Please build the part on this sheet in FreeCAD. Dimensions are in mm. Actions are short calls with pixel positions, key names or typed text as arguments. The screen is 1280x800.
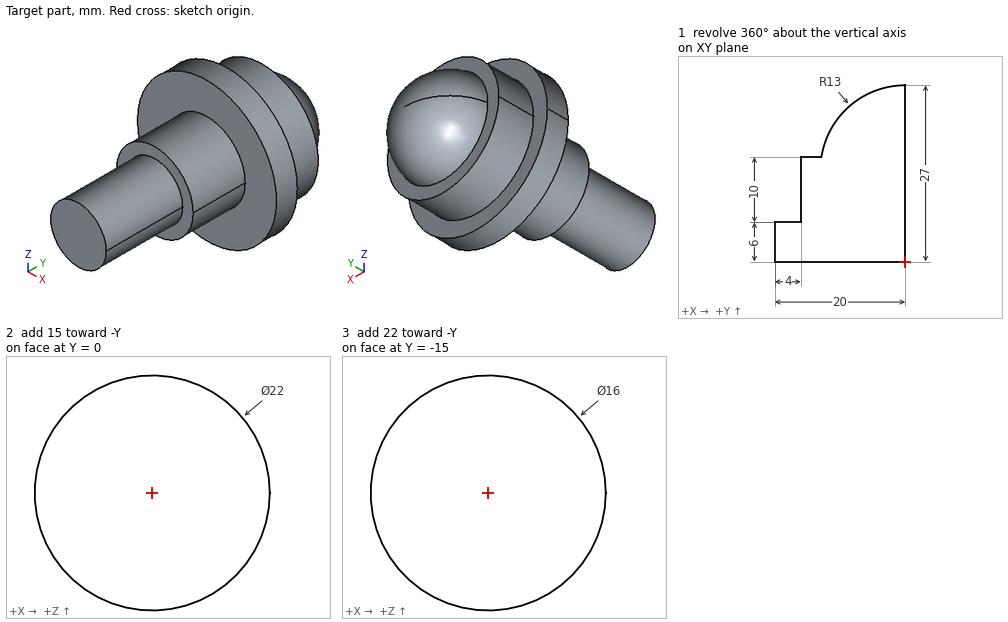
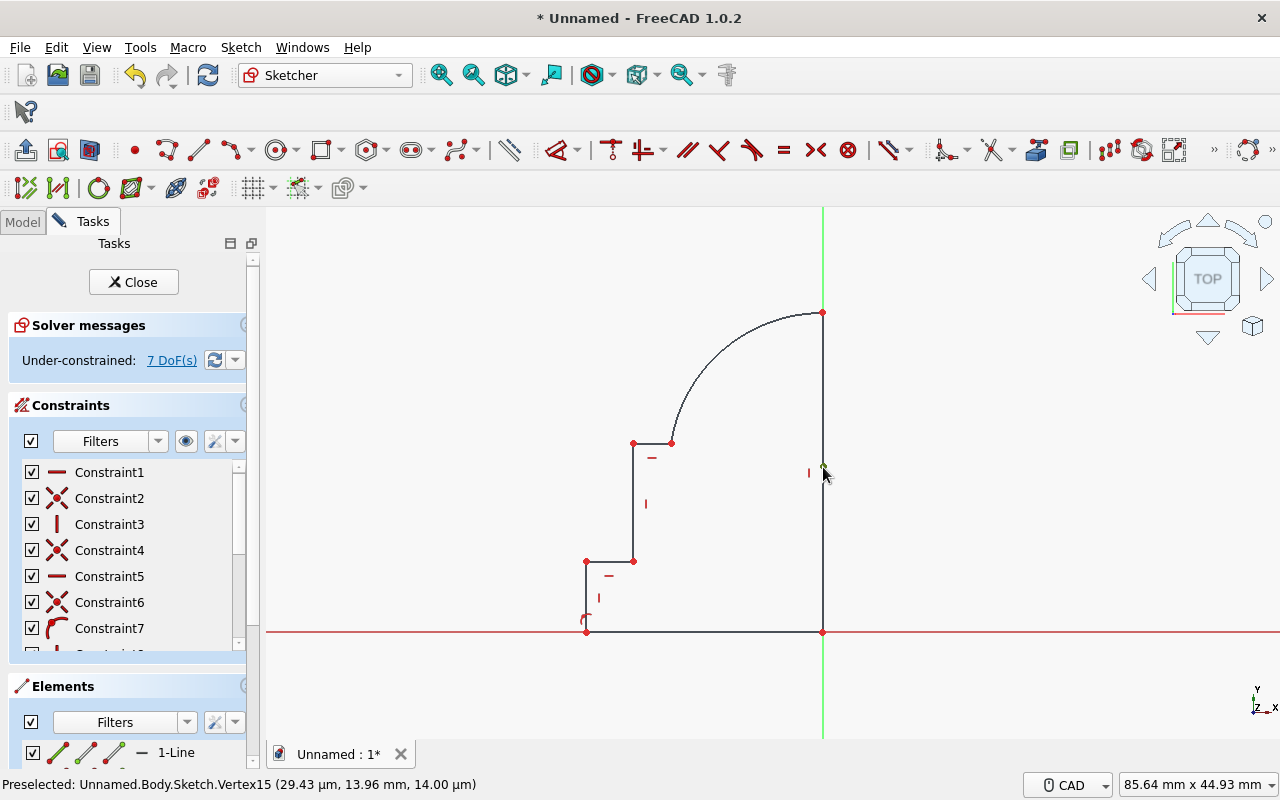
click(823, 677)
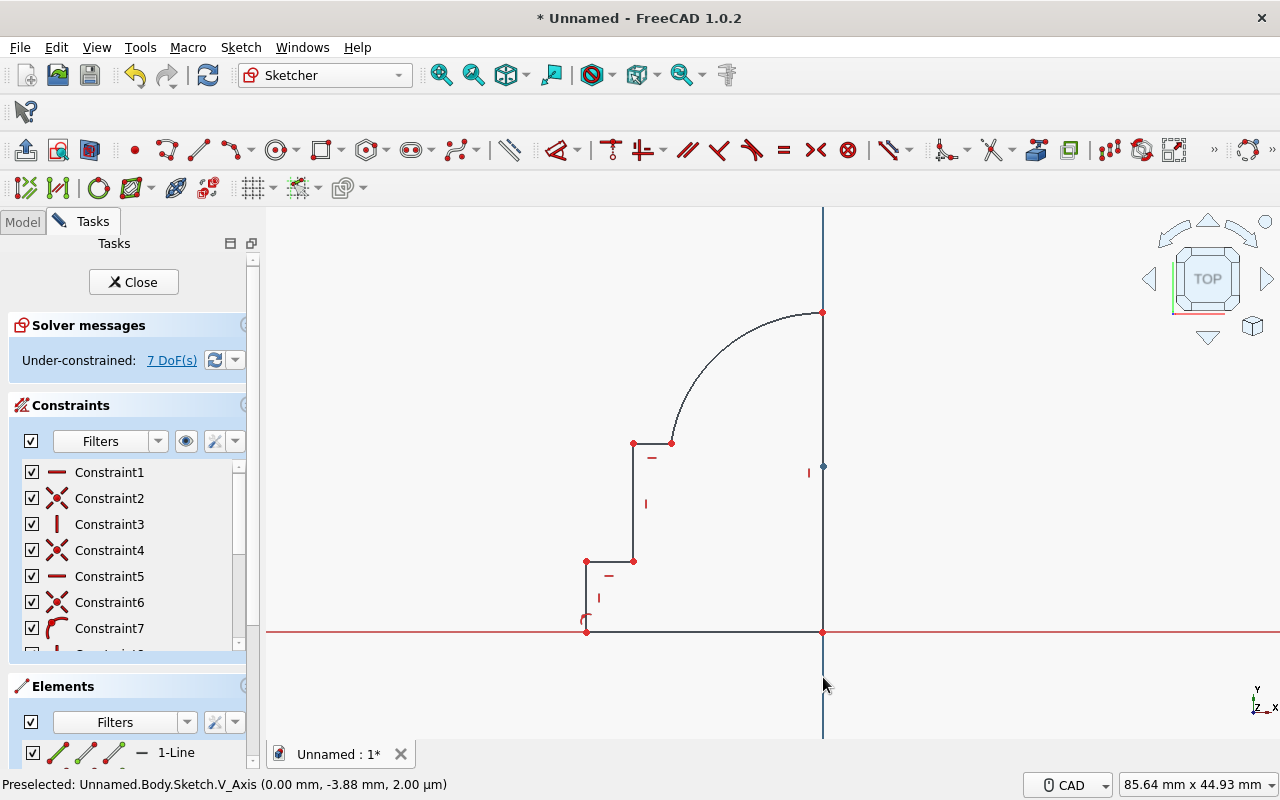
click(612, 150)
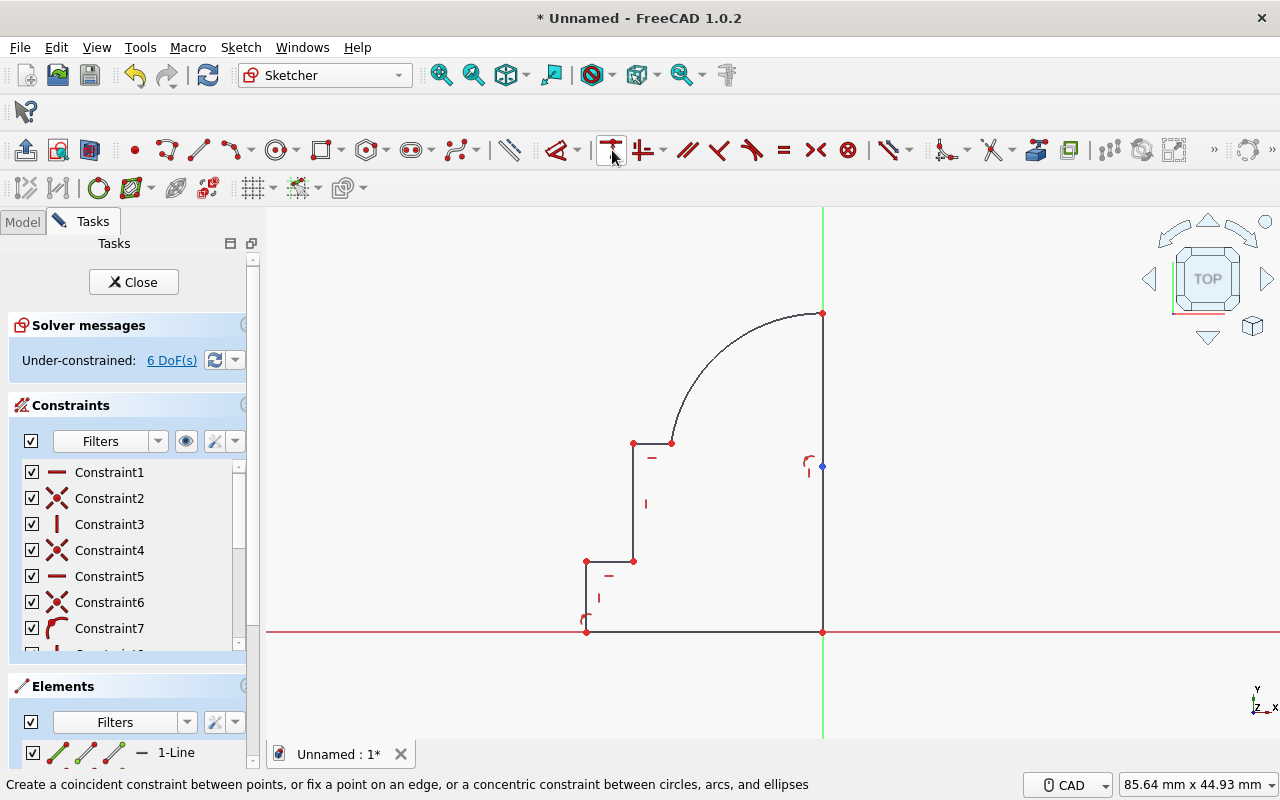
click(556, 150)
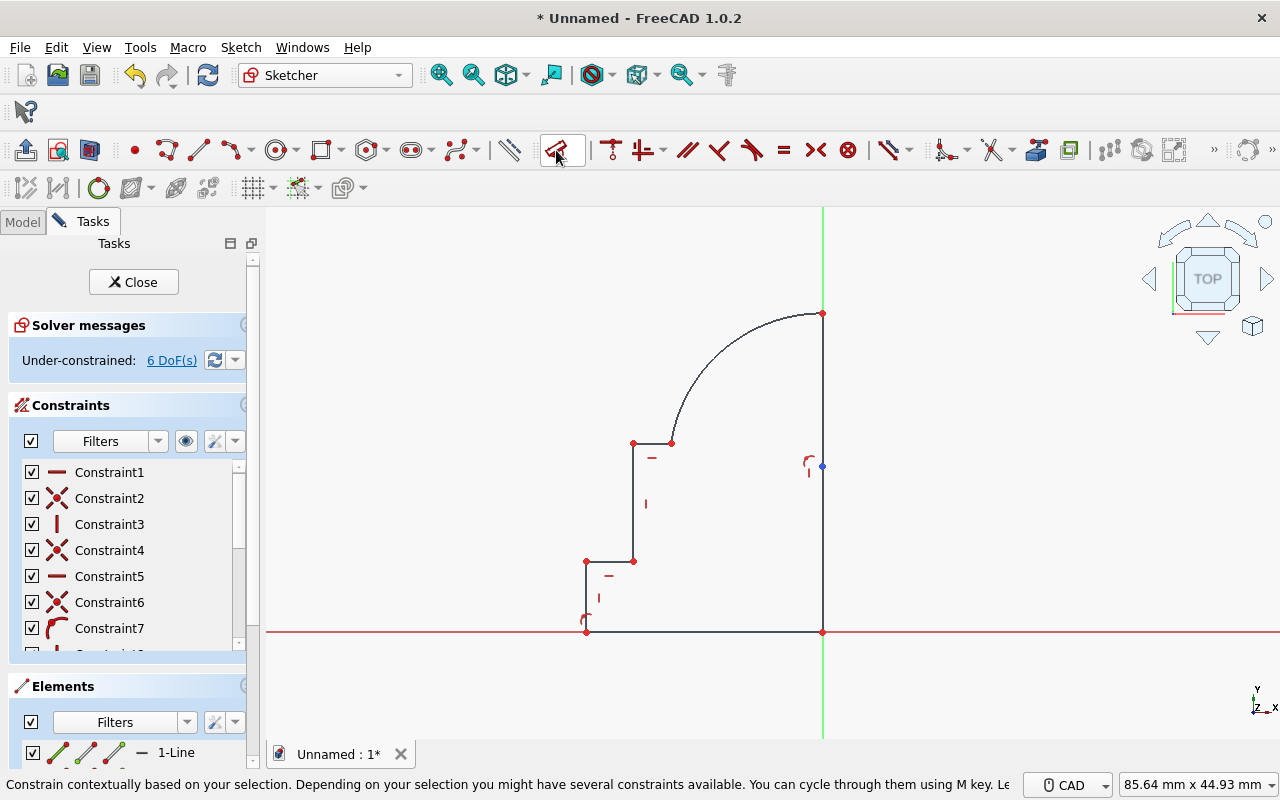
click(759, 327)
click(746, 298)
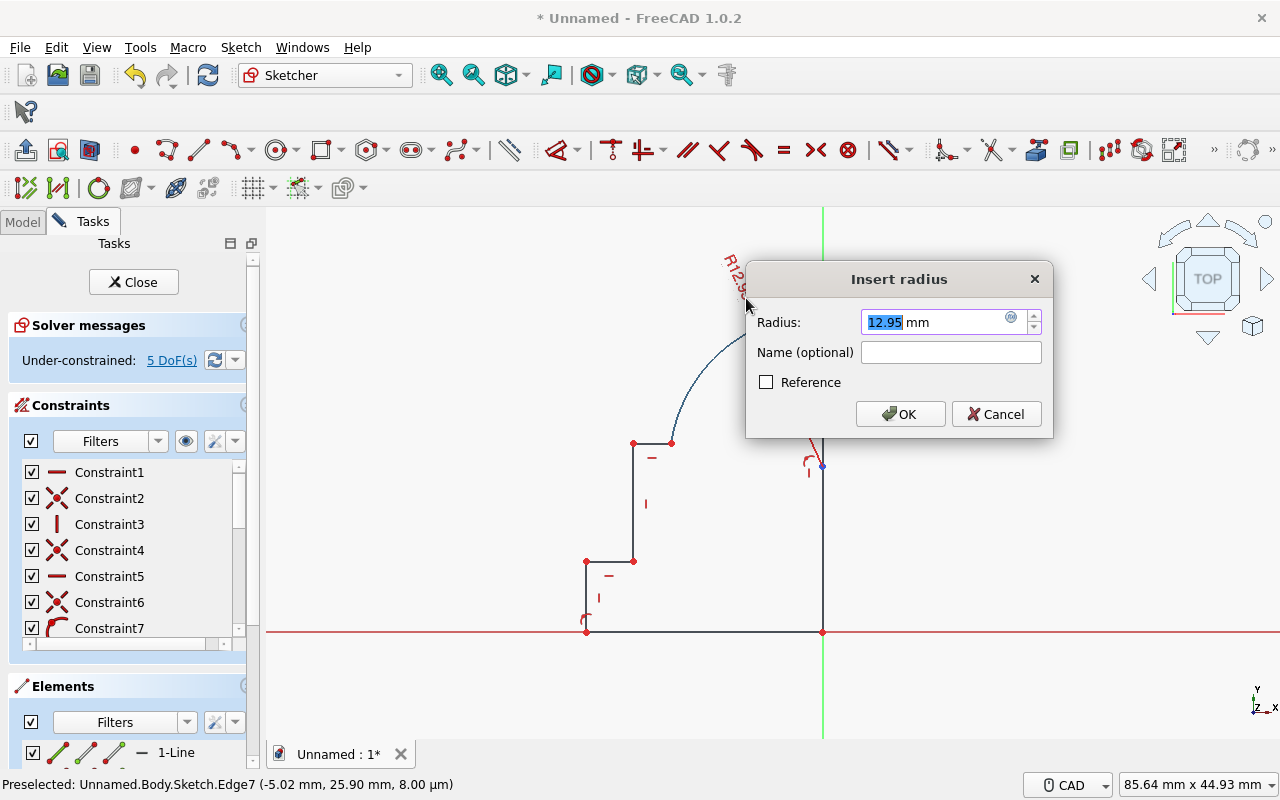
text(13)
key(Return)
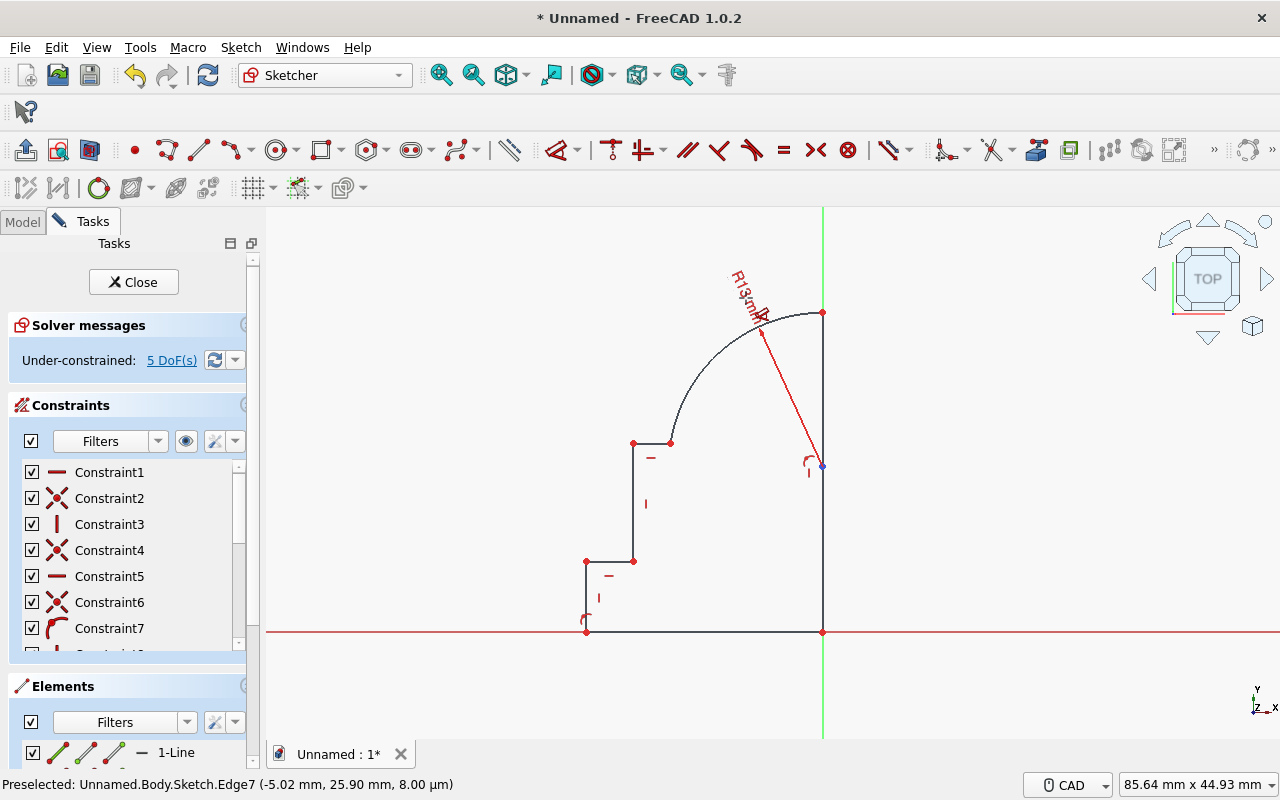
click(619, 562)
click(609, 596)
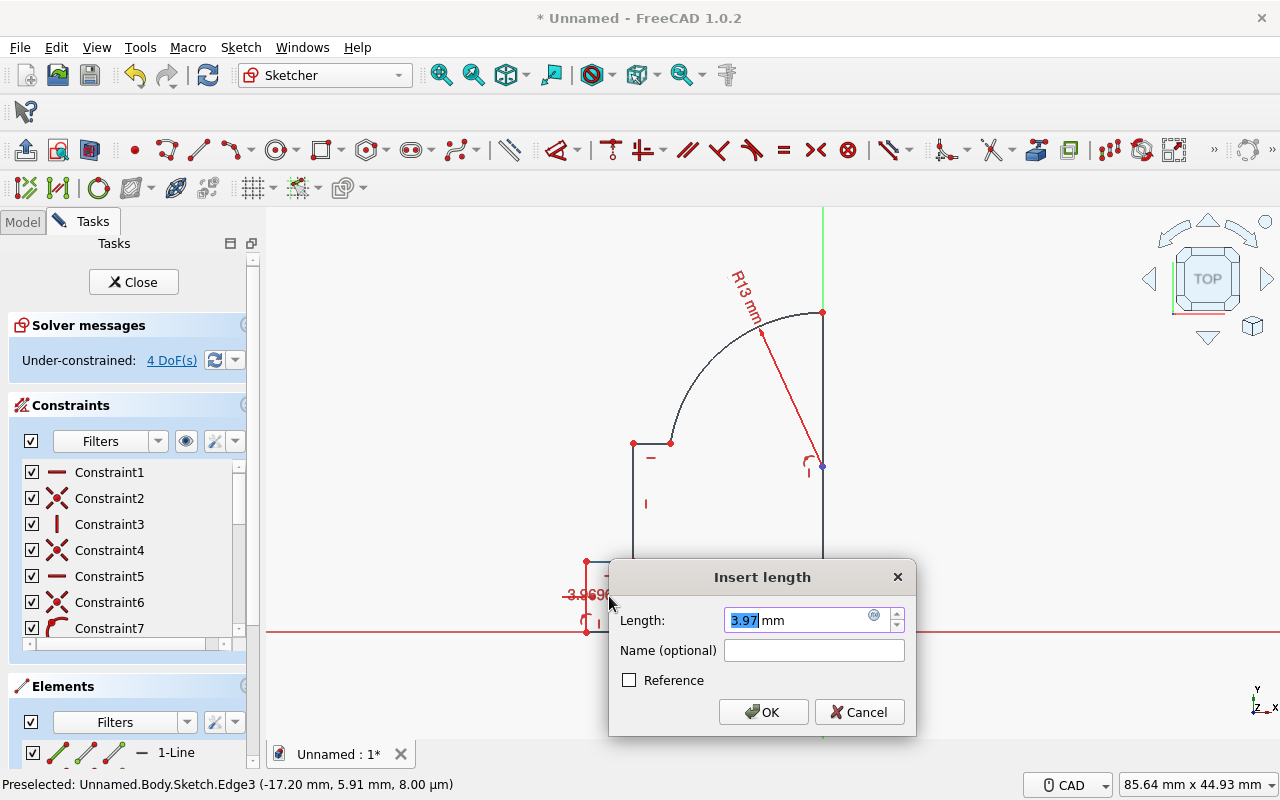
text(4)
key(Return)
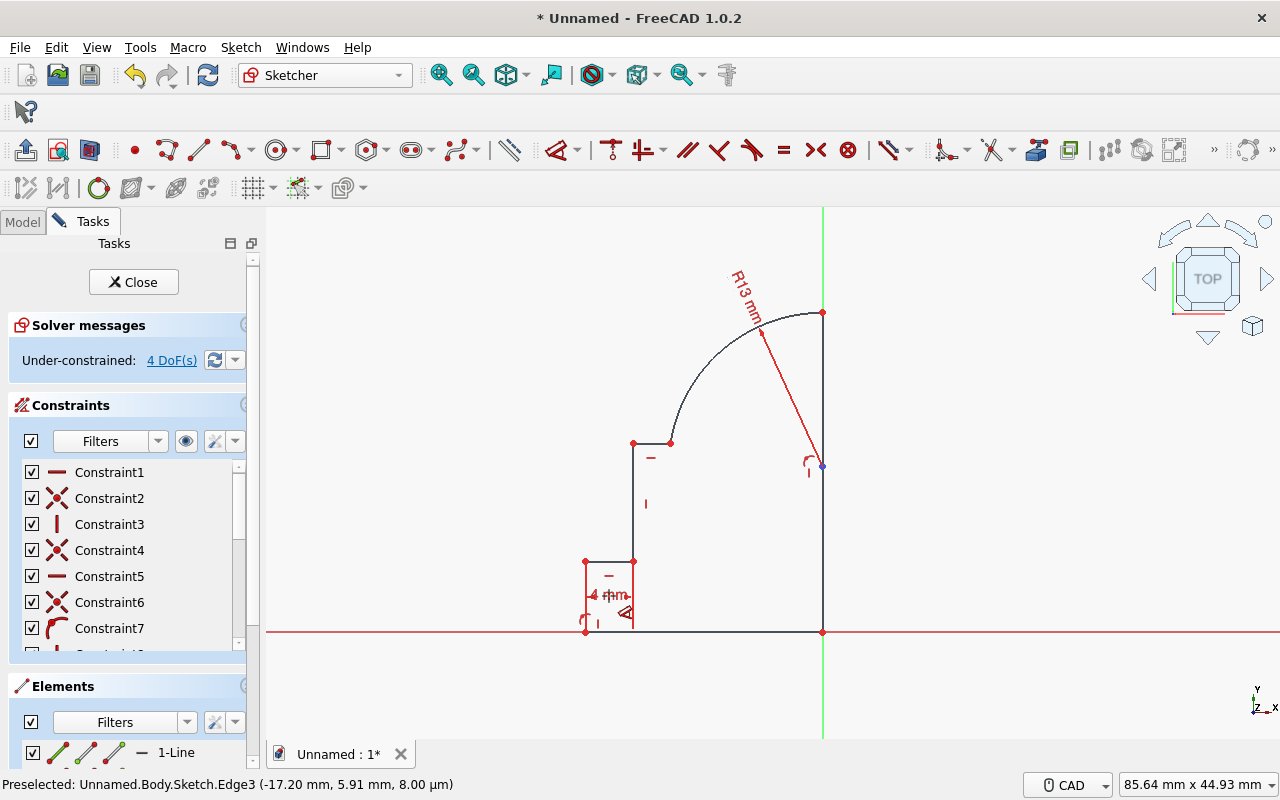
click(586, 583)
click(552, 573)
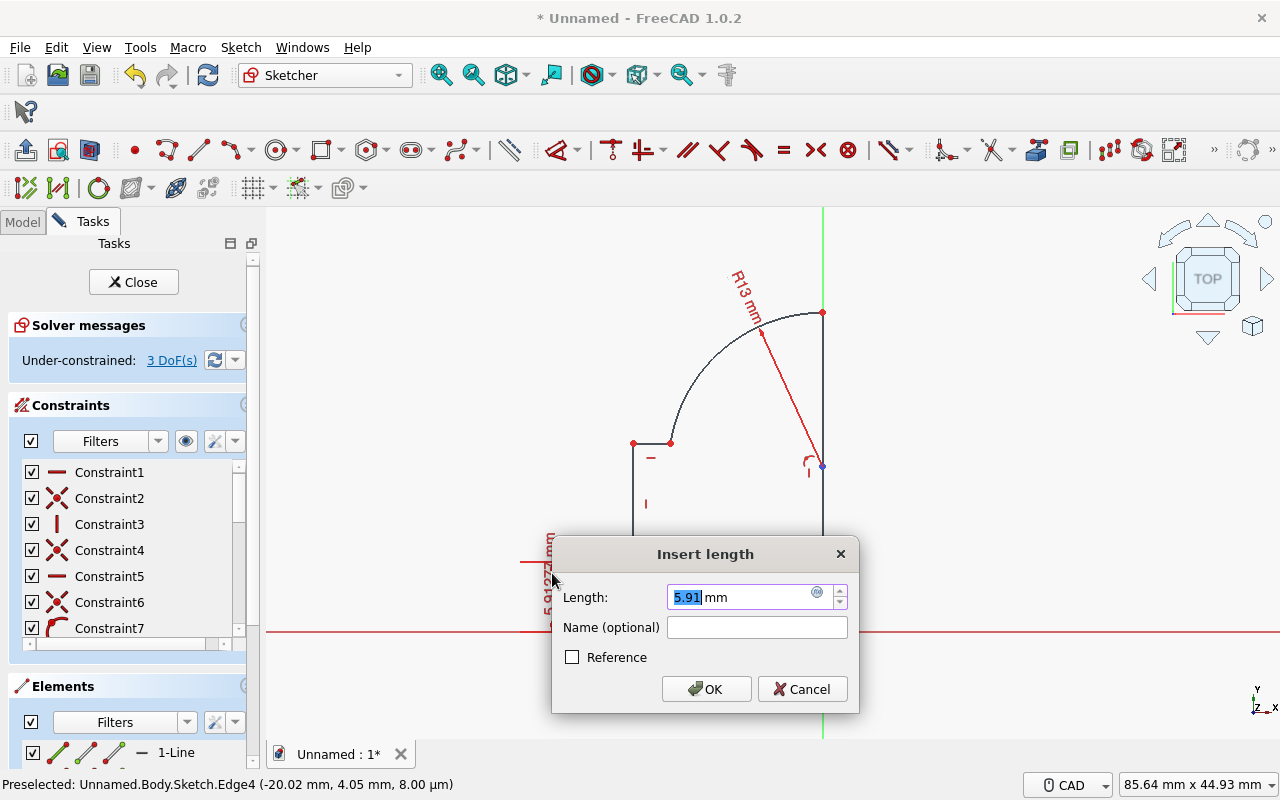
text(6)
key(Return)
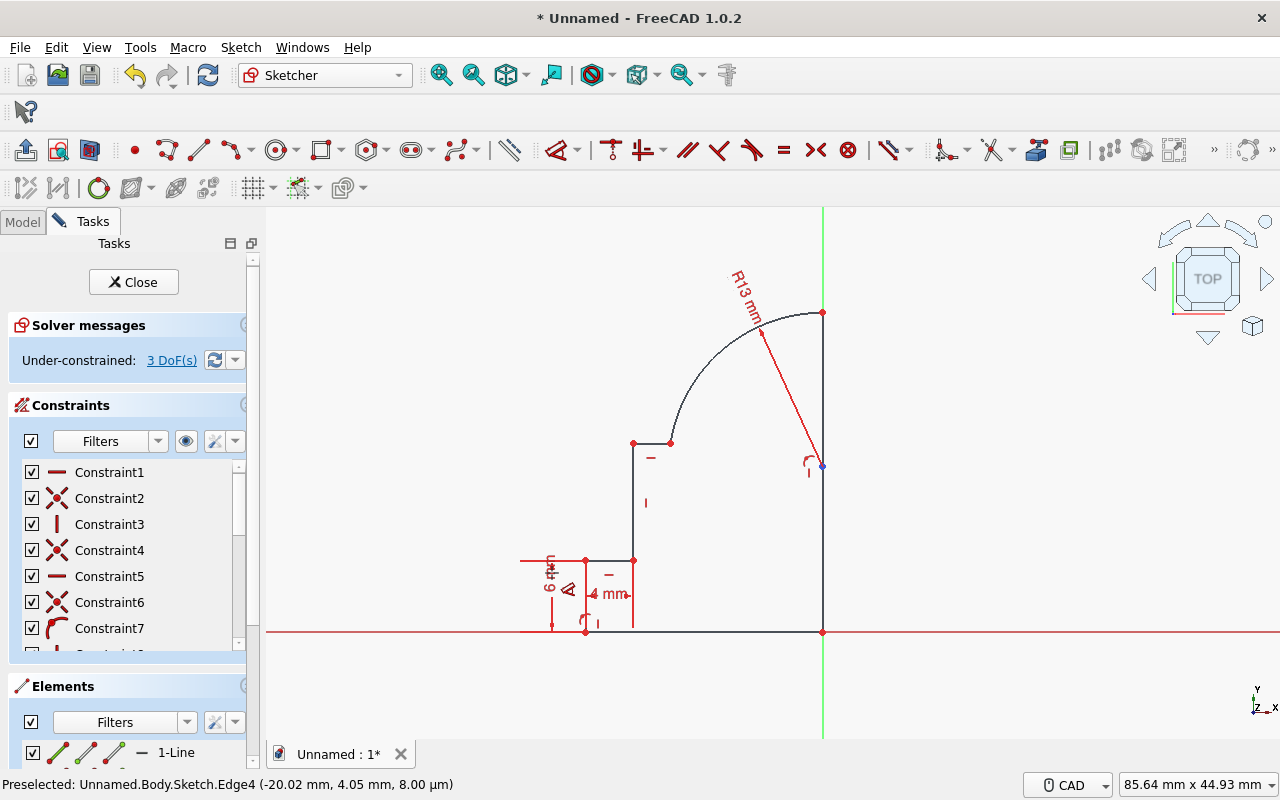
click(633, 479)
click(599, 502)